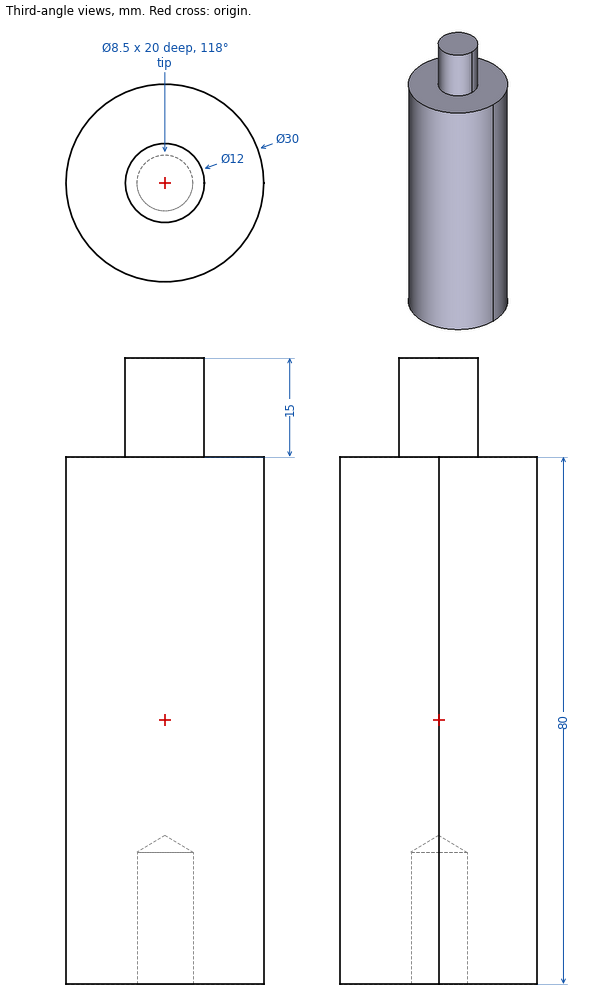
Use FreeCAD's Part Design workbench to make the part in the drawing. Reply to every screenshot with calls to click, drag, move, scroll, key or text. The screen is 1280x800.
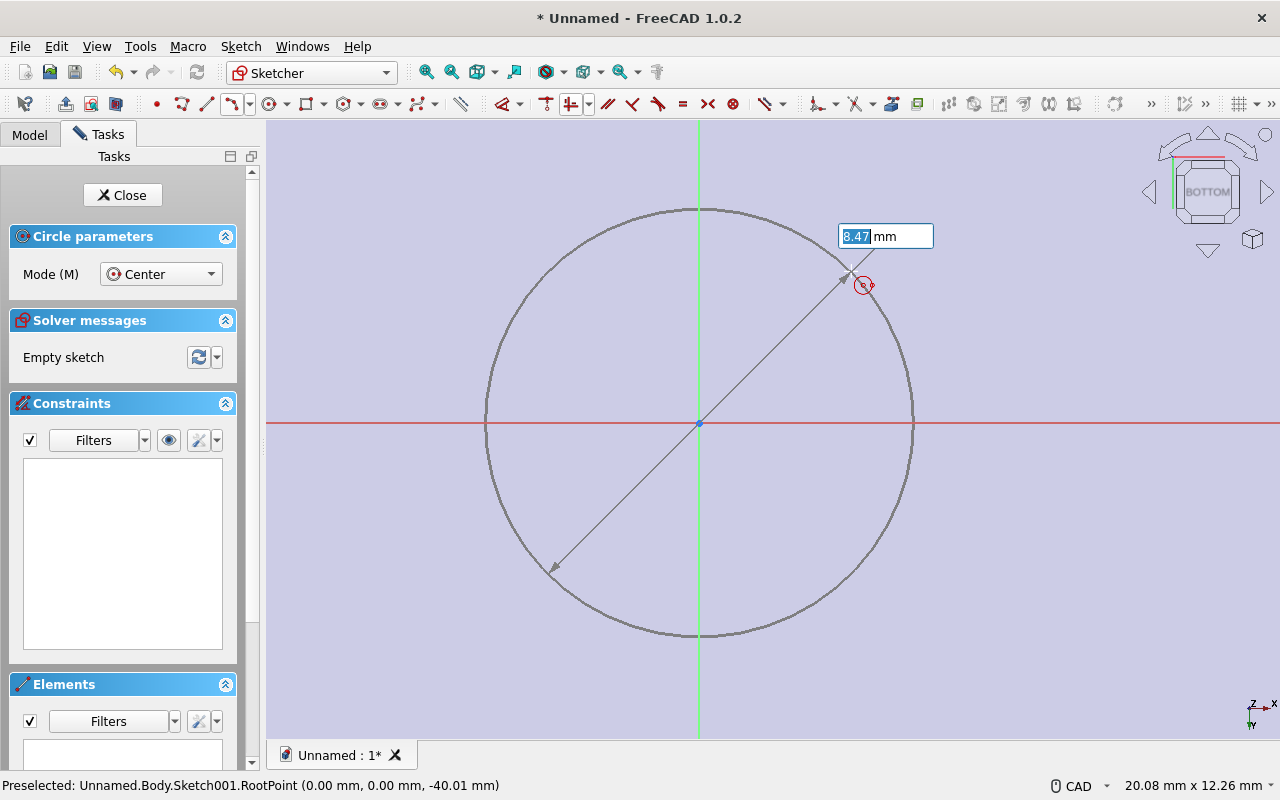
text(8.5)
key(Return)
key(Escape)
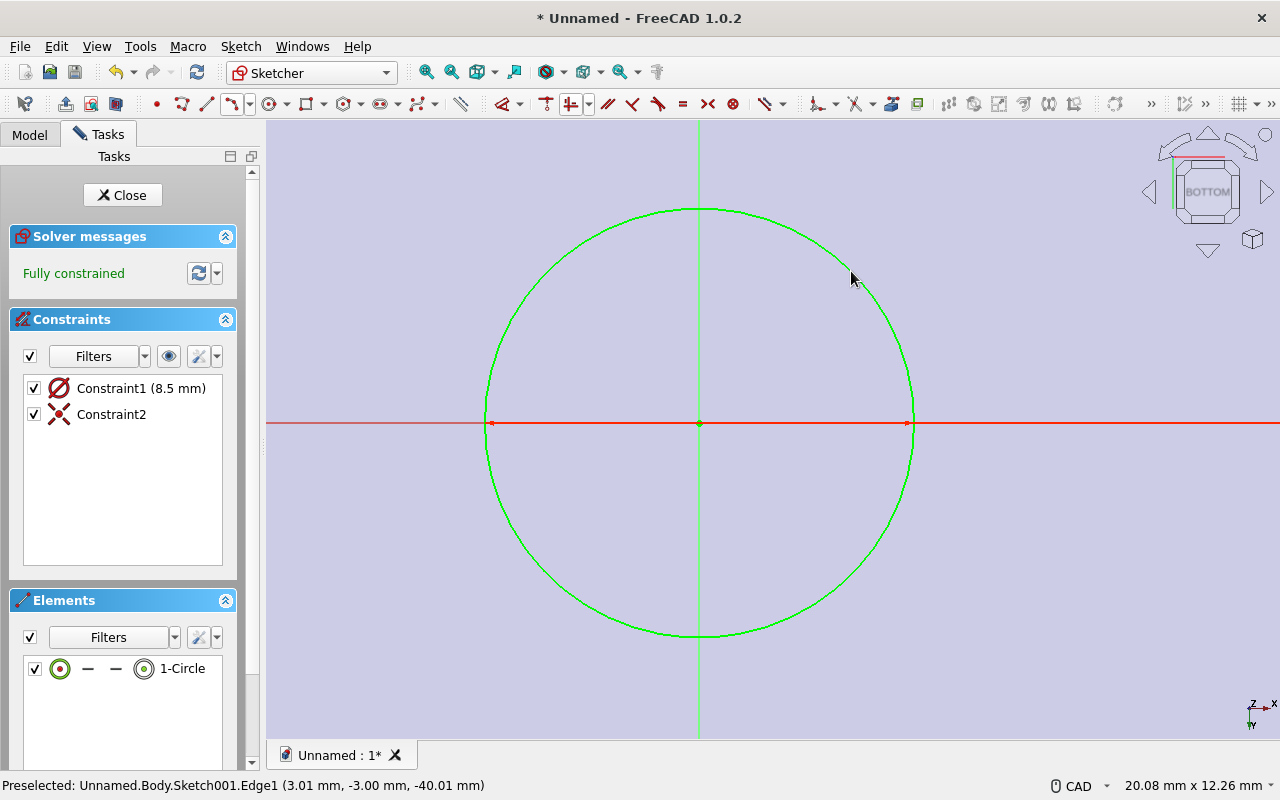
click(123, 195)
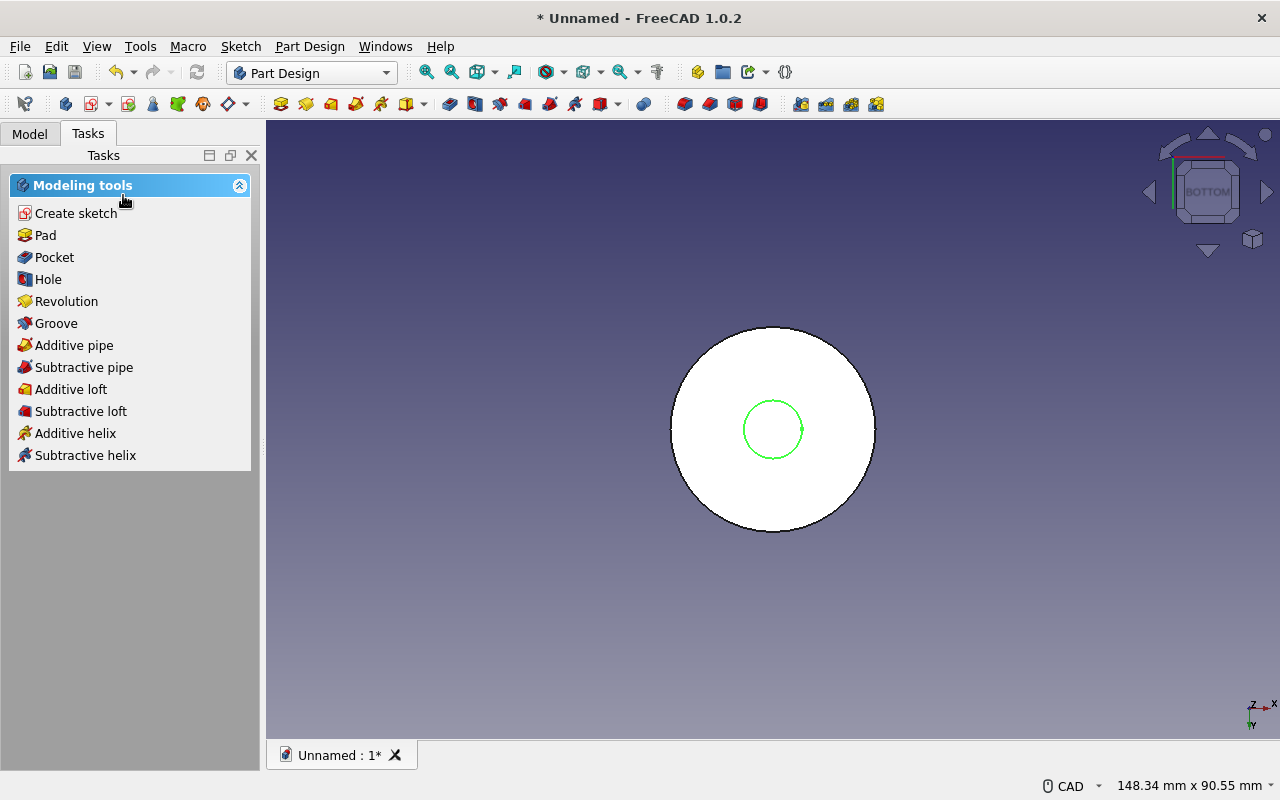
click(475, 104)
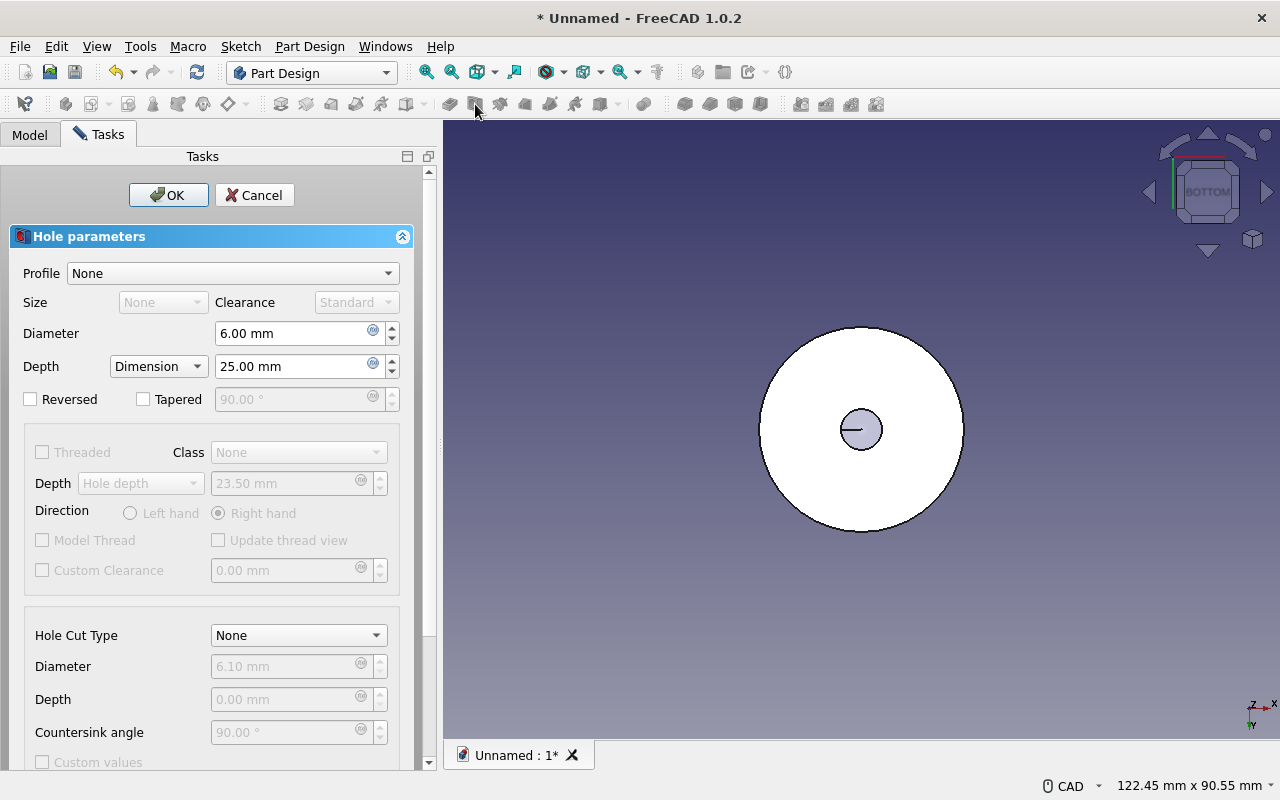
triple_click(300, 334)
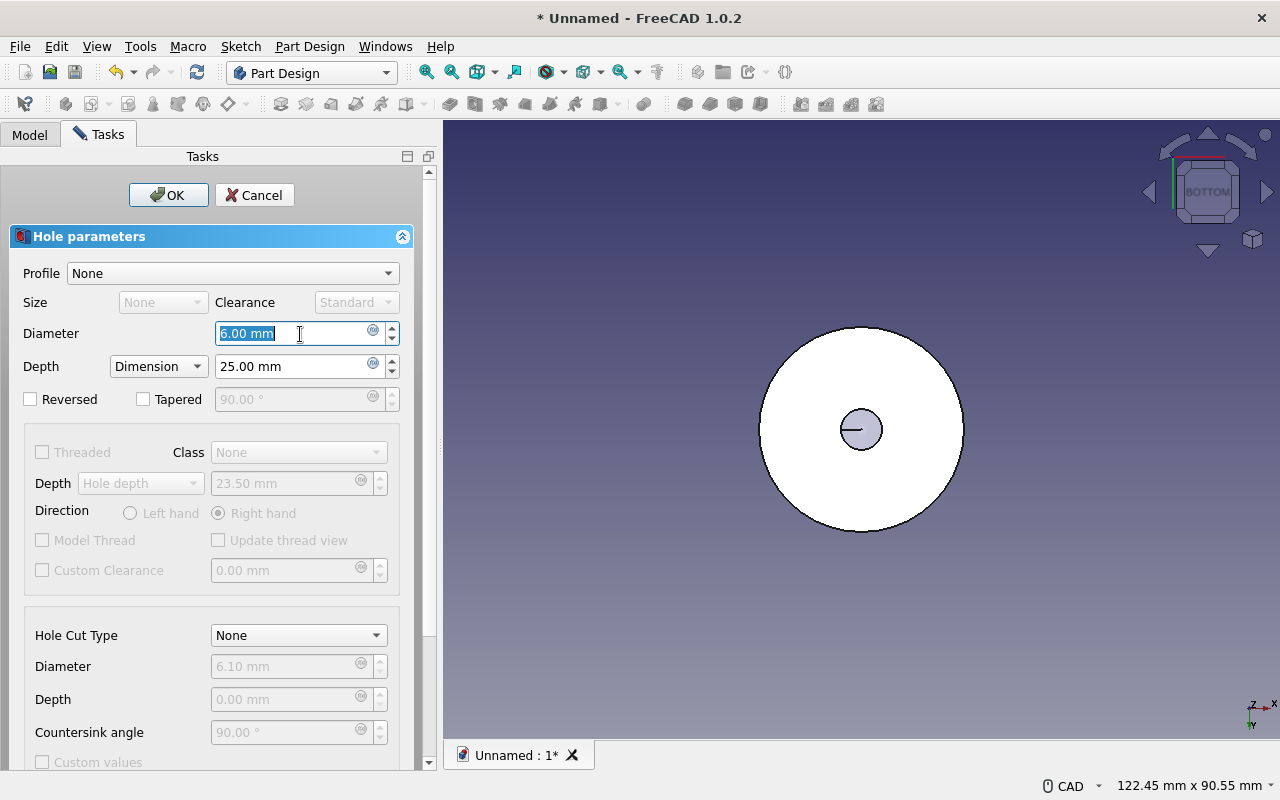
text(8.5)
key(Tab)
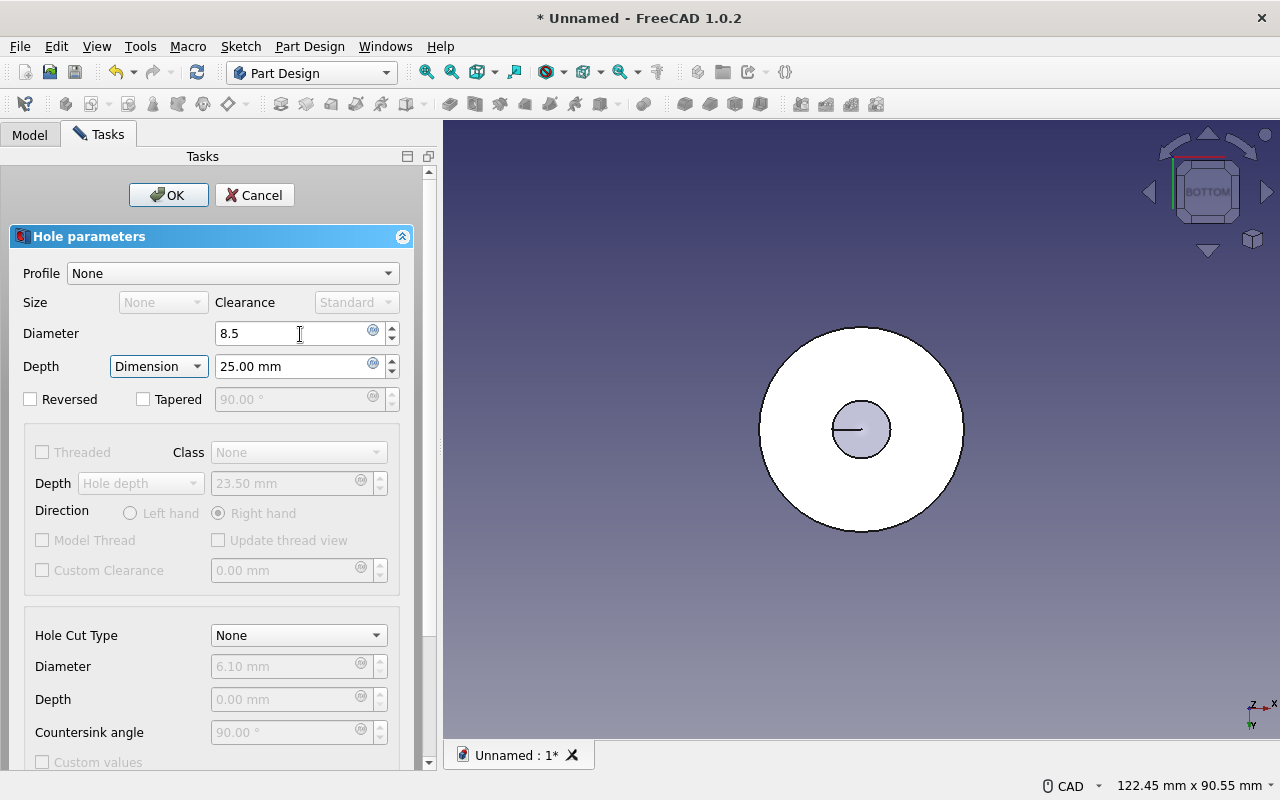
triple_click(300, 366)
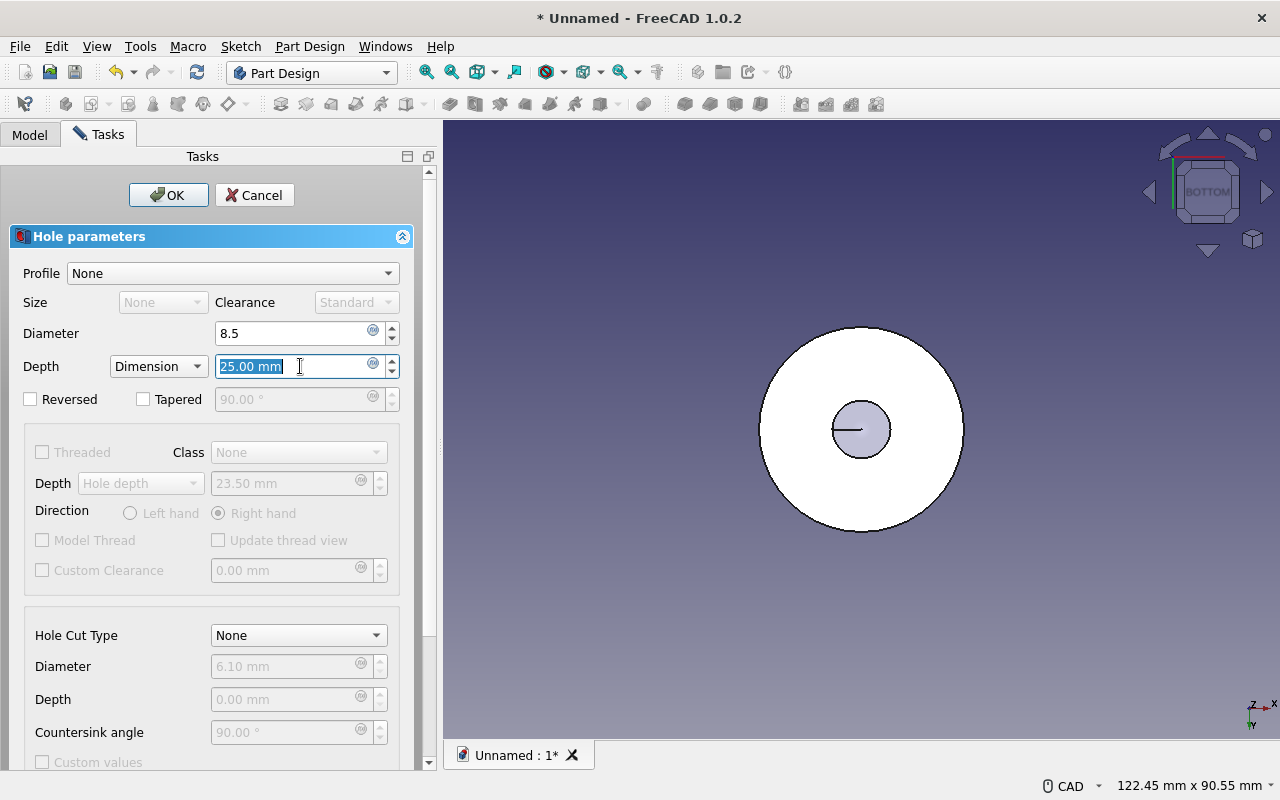
text(20)
key(Tab)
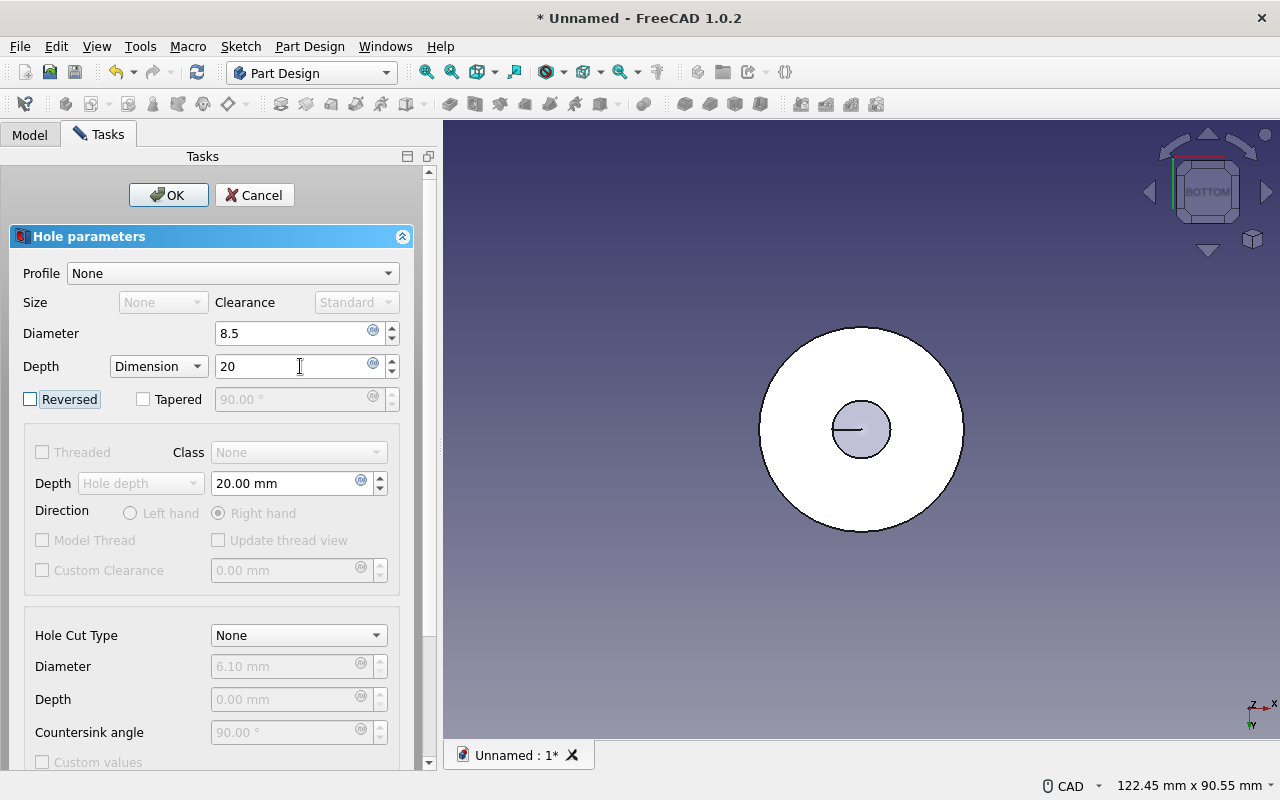
click(169, 195)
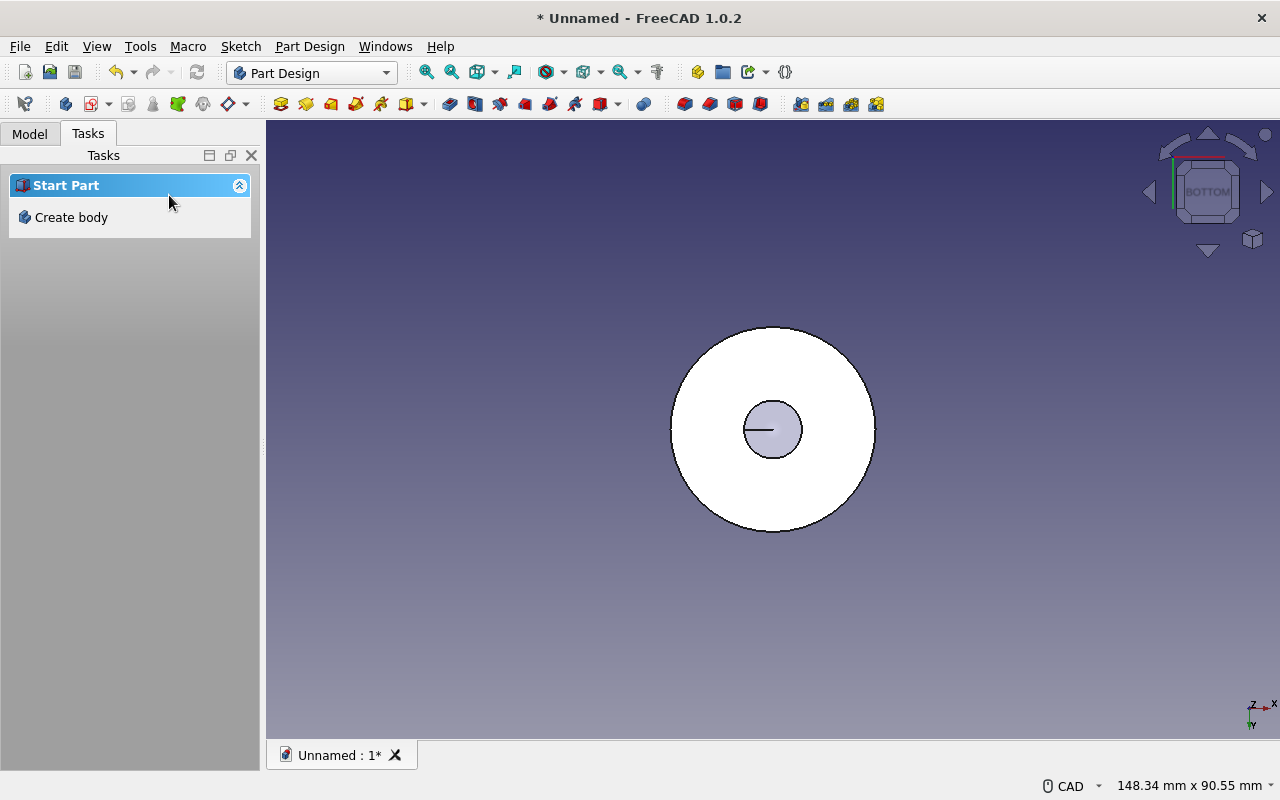
click(427, 72)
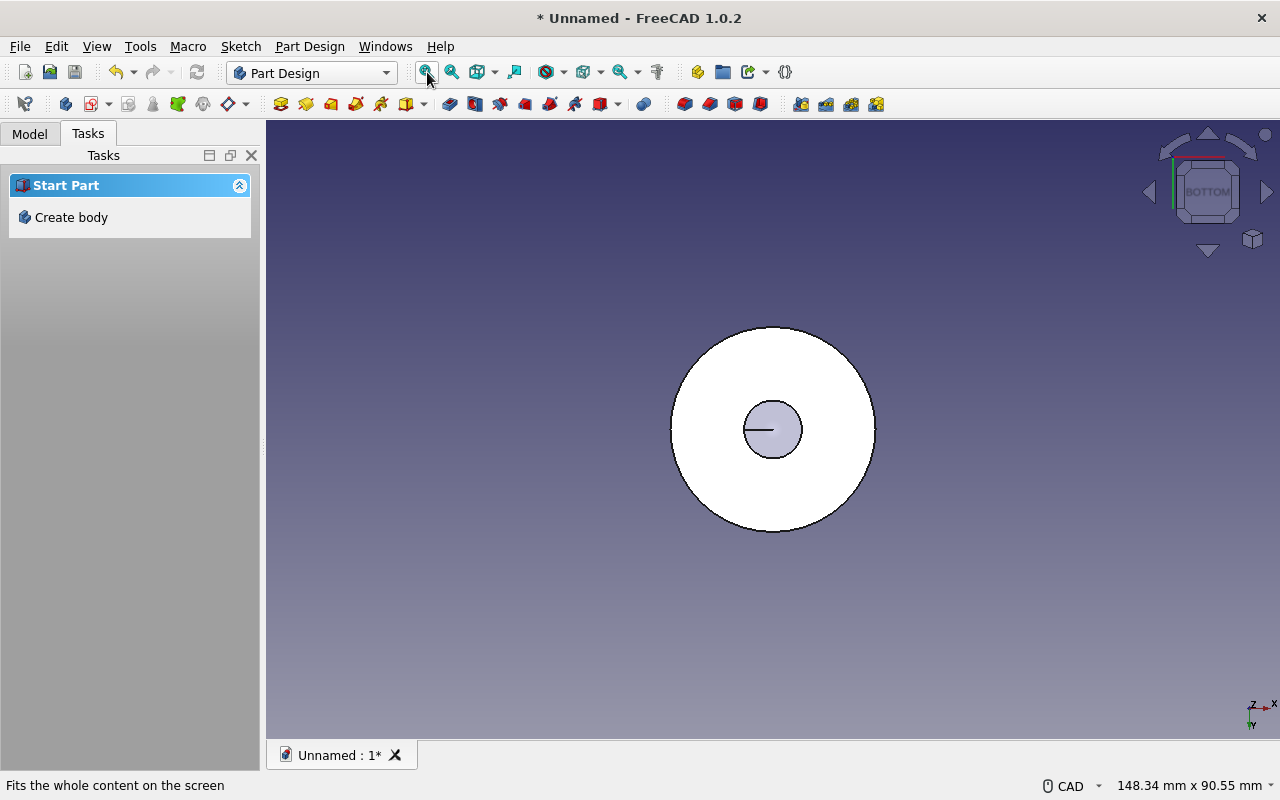
key(0)